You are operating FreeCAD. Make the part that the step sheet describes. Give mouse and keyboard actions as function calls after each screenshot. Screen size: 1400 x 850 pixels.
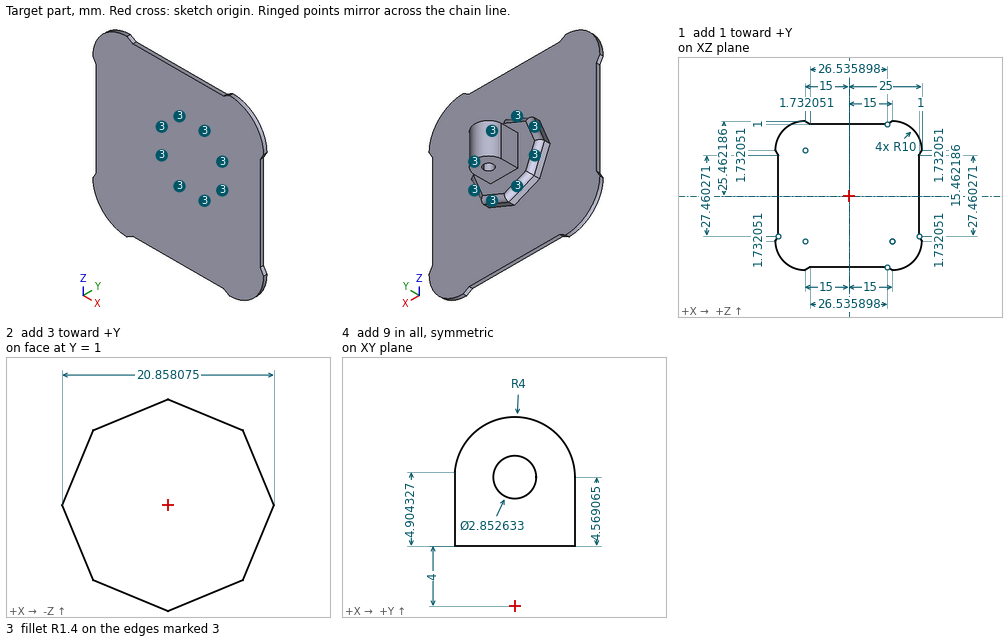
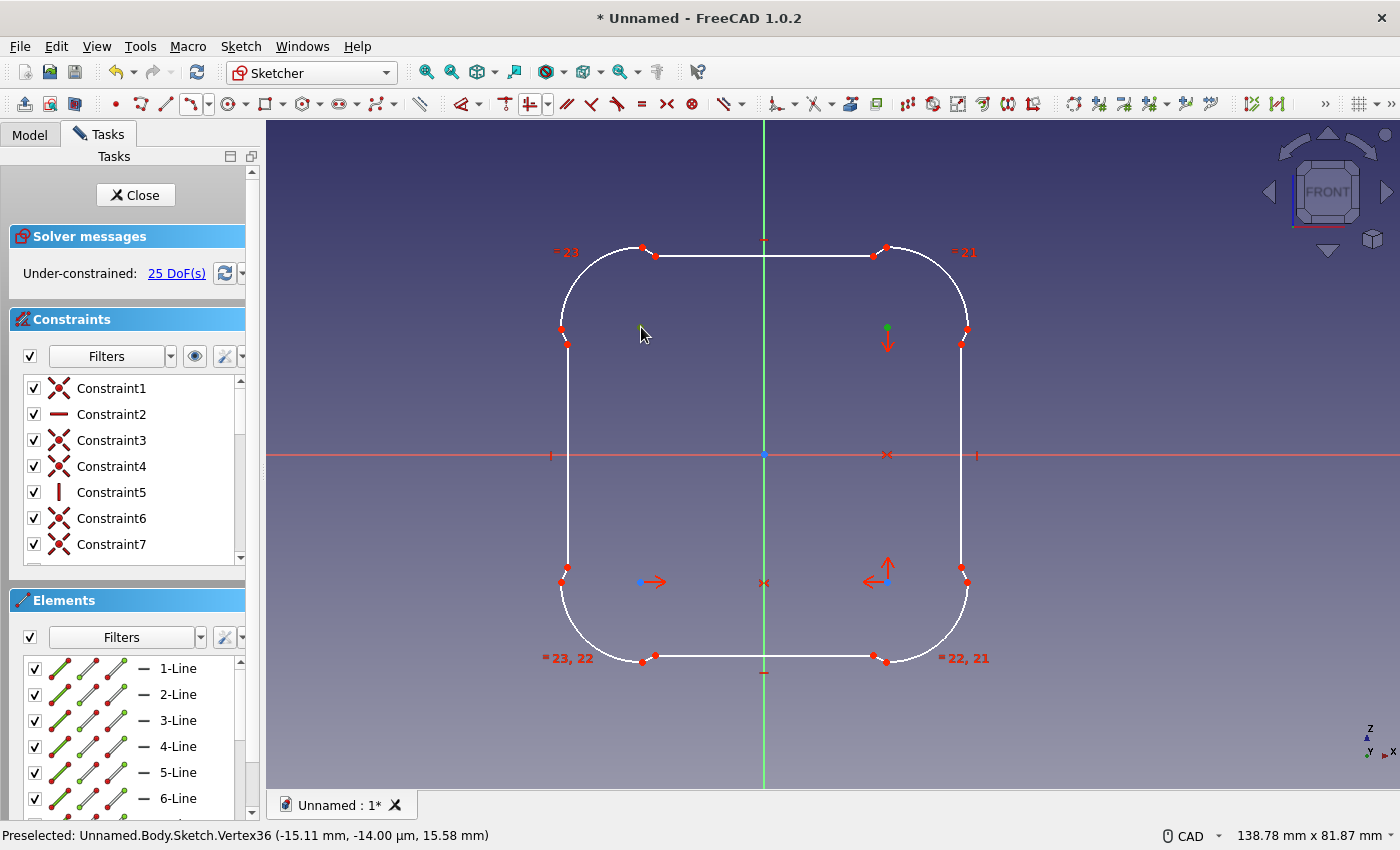
click(764, 717)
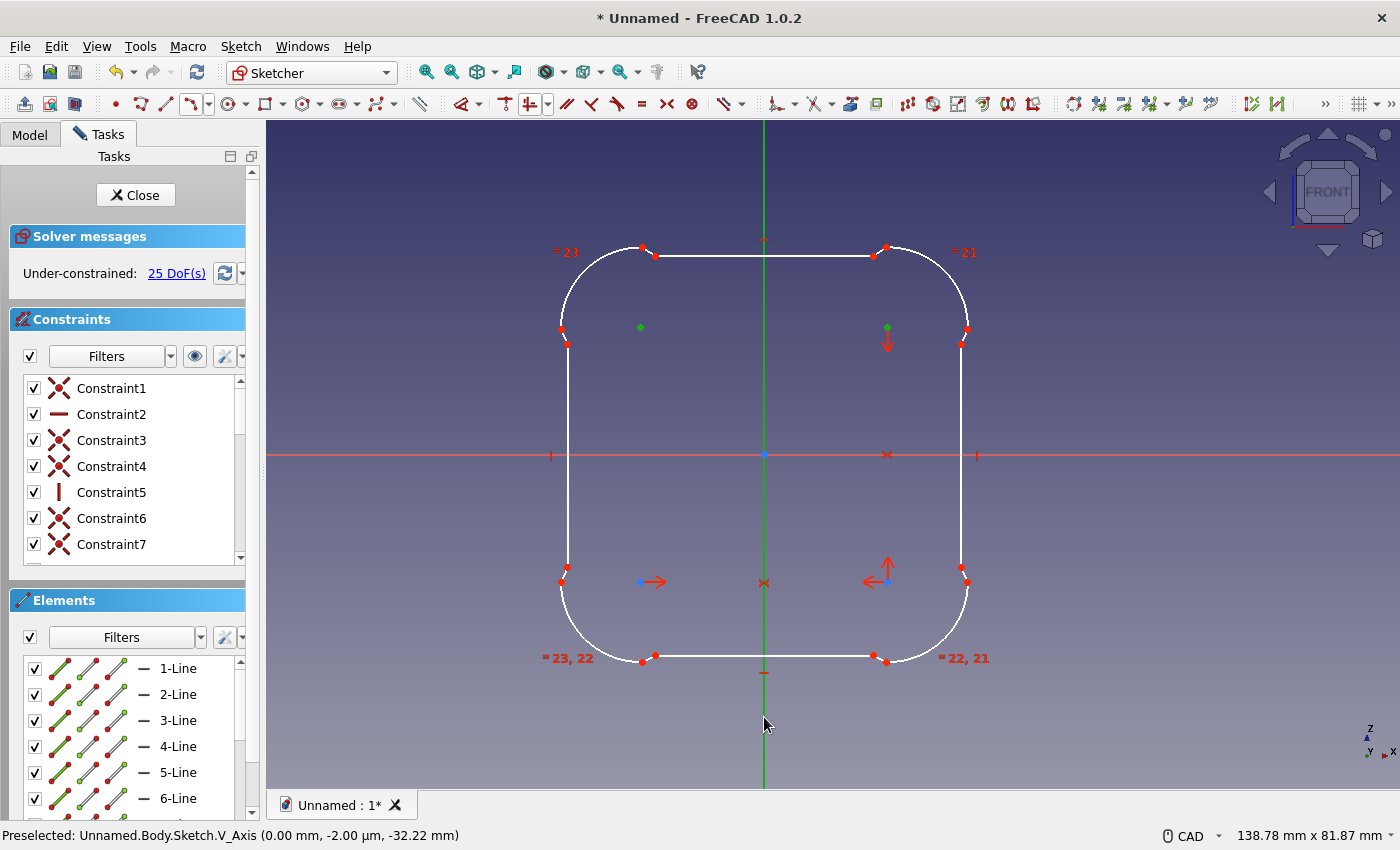
click(667, 104)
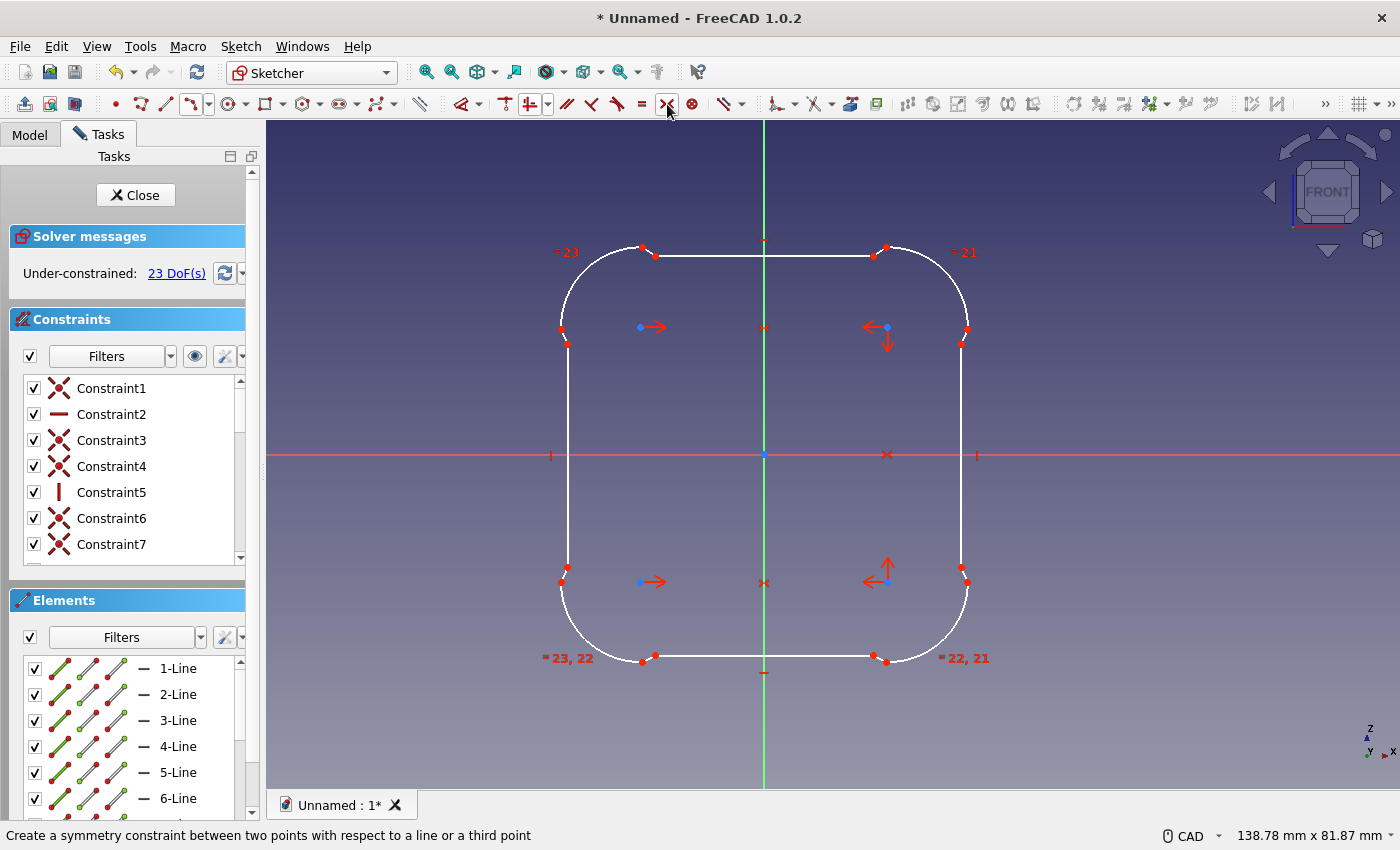
click(873, 256)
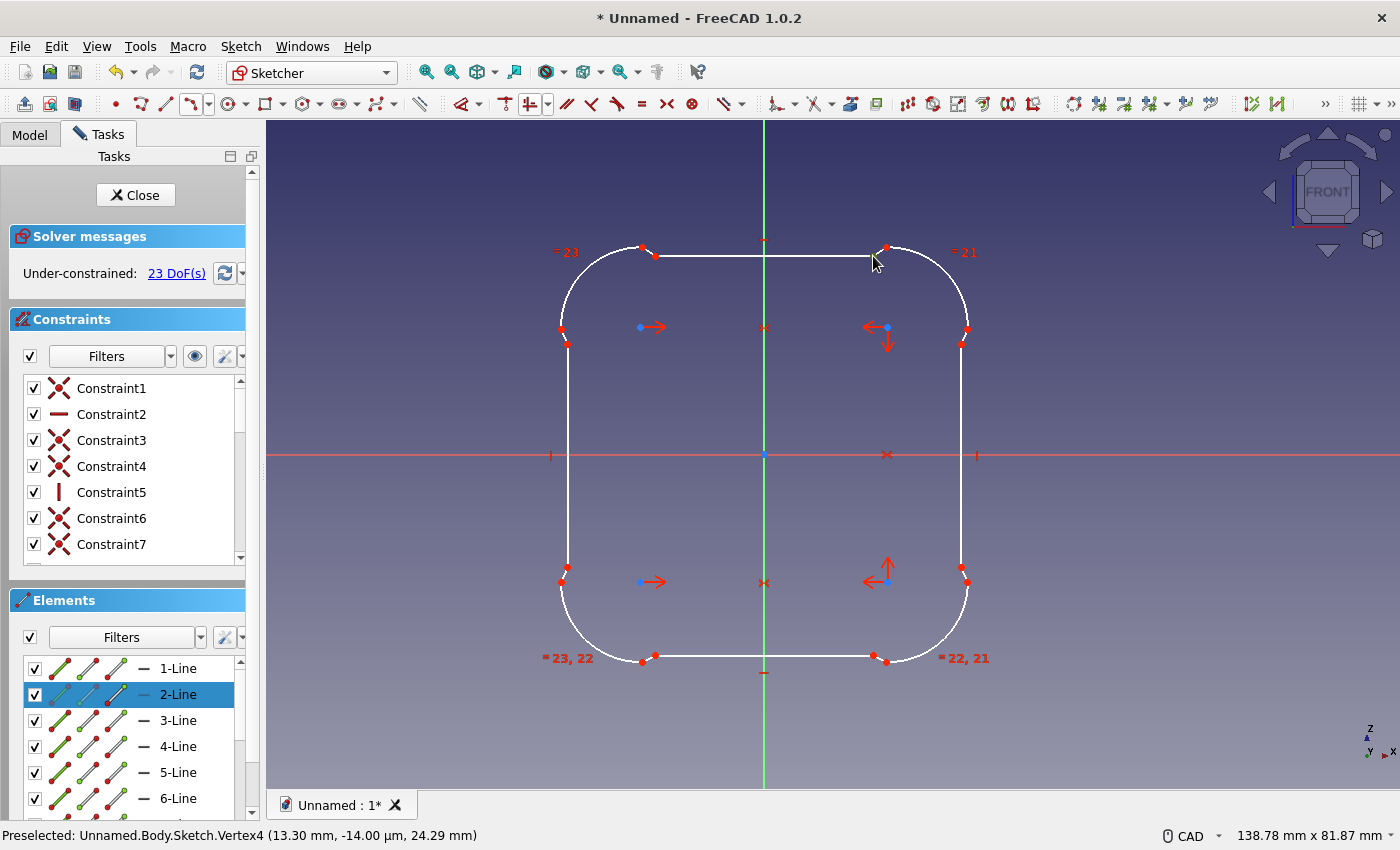
click(873, 656)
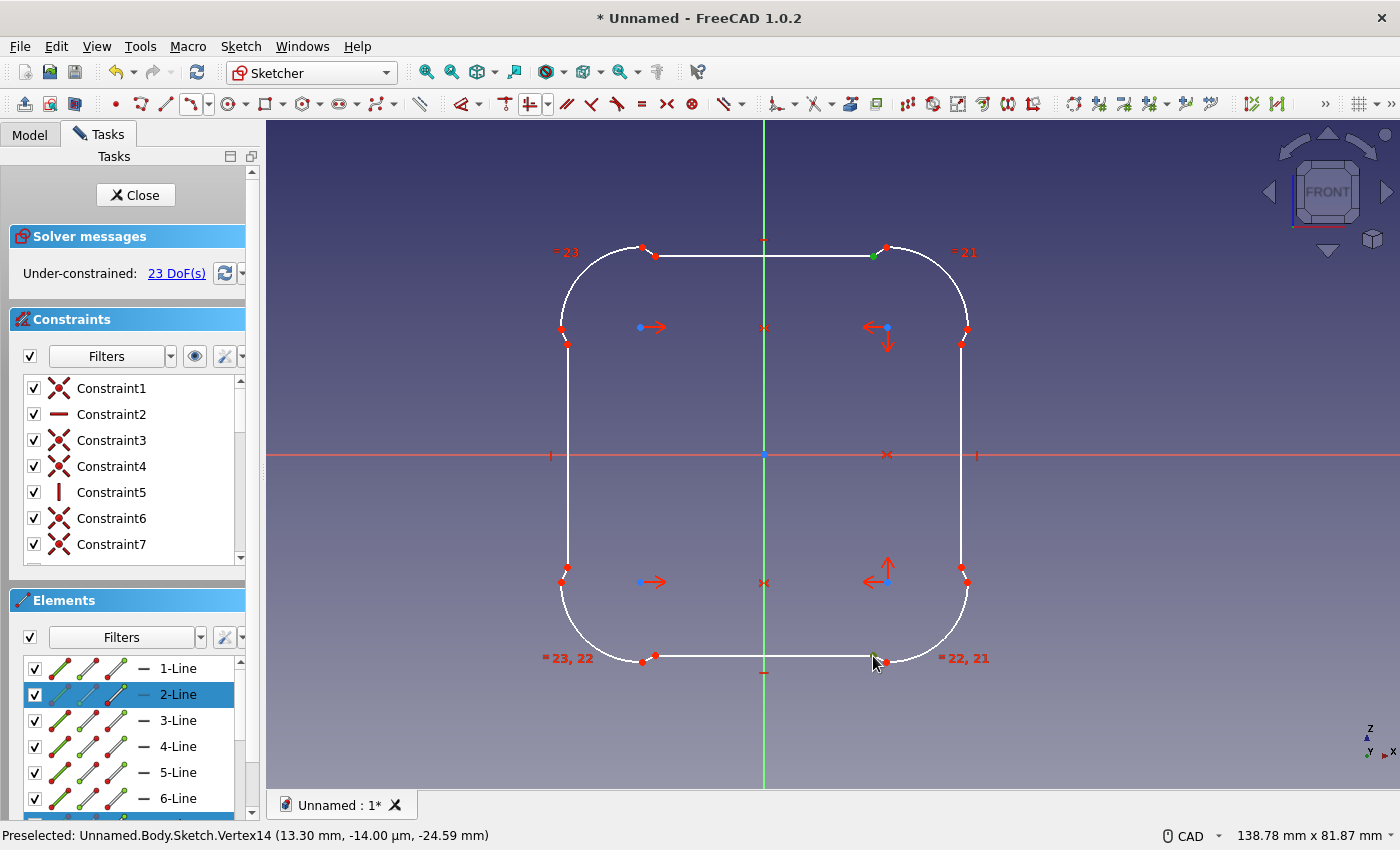
click(361, 455)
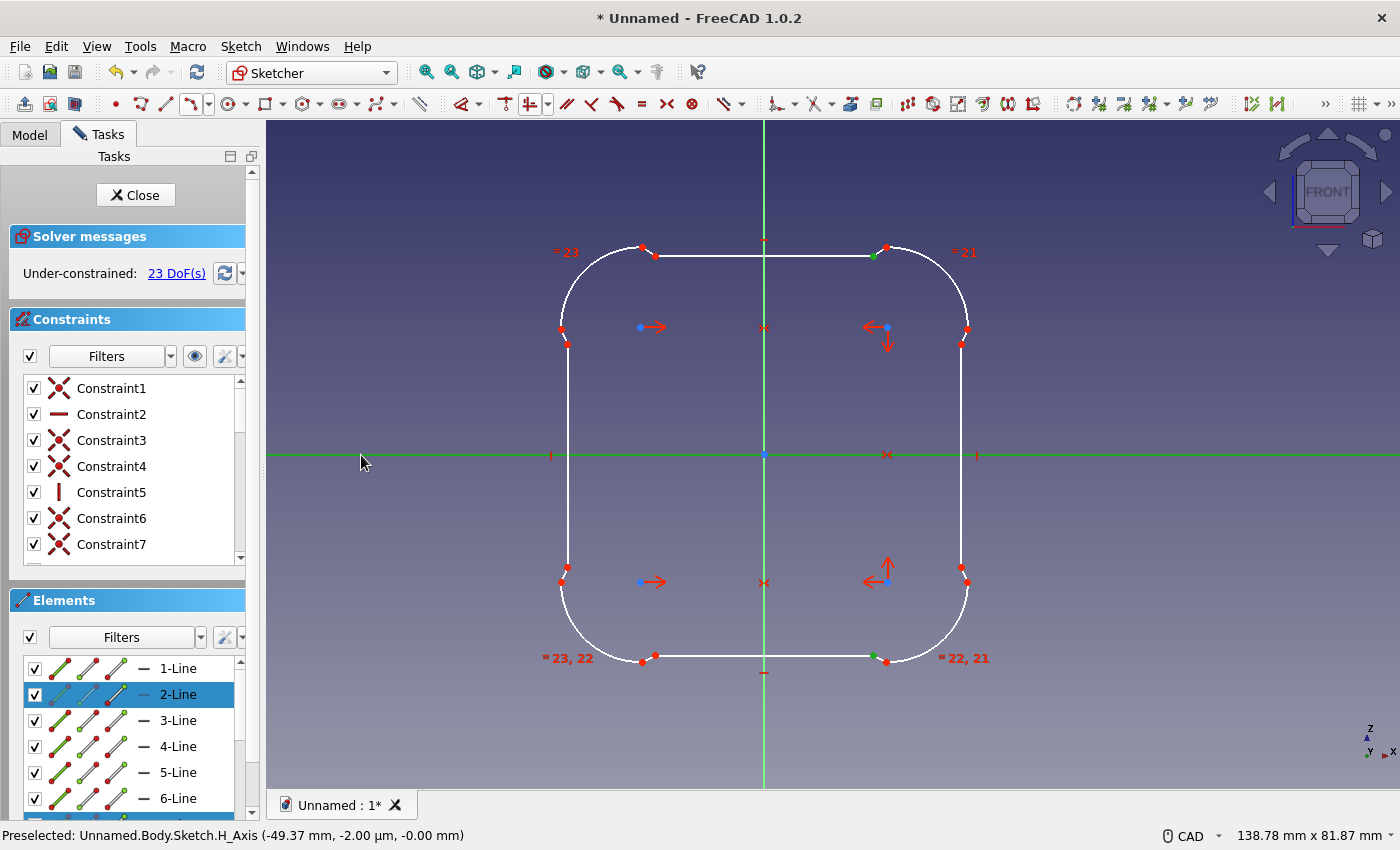
click(667, 104)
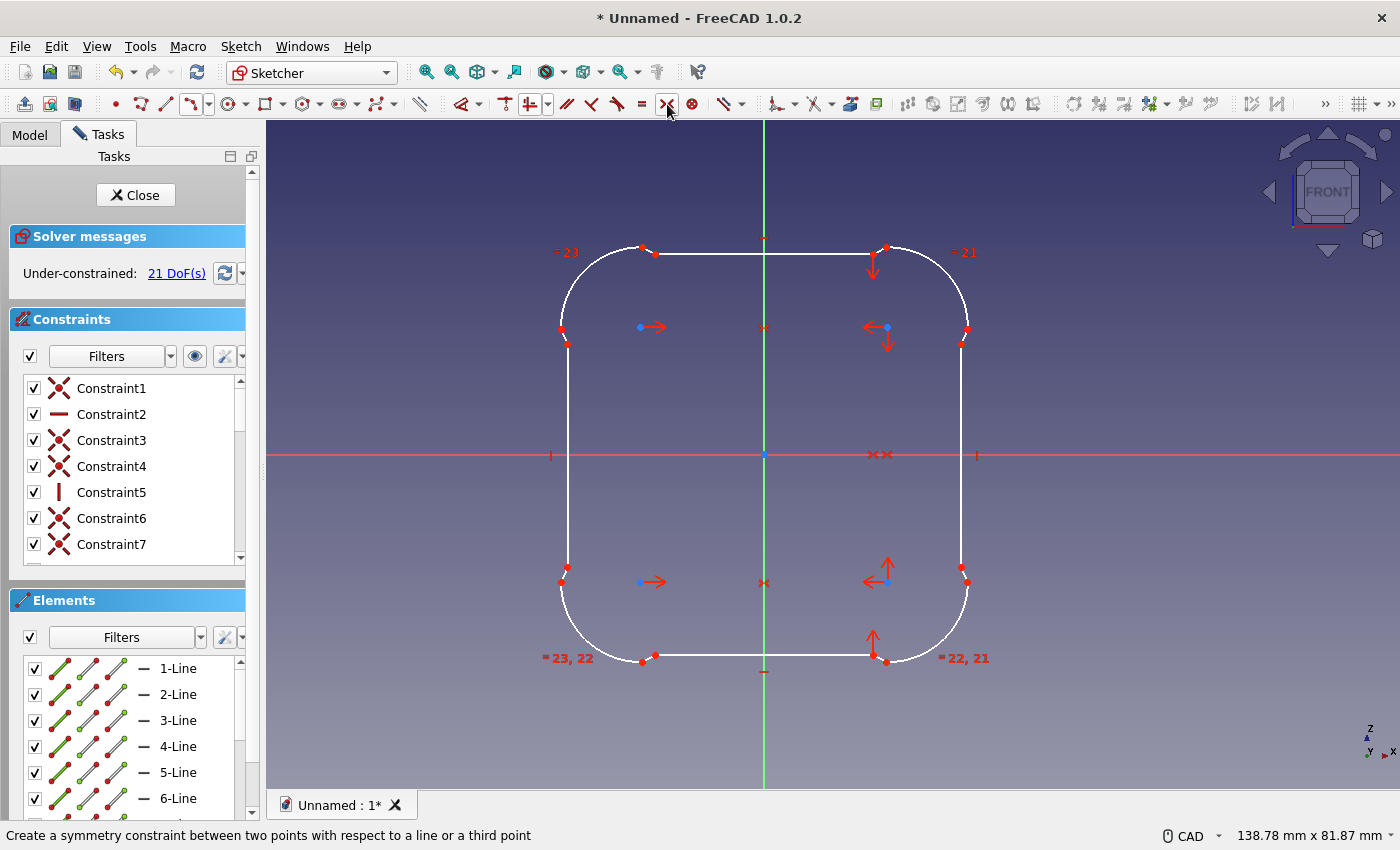
click(961, 568)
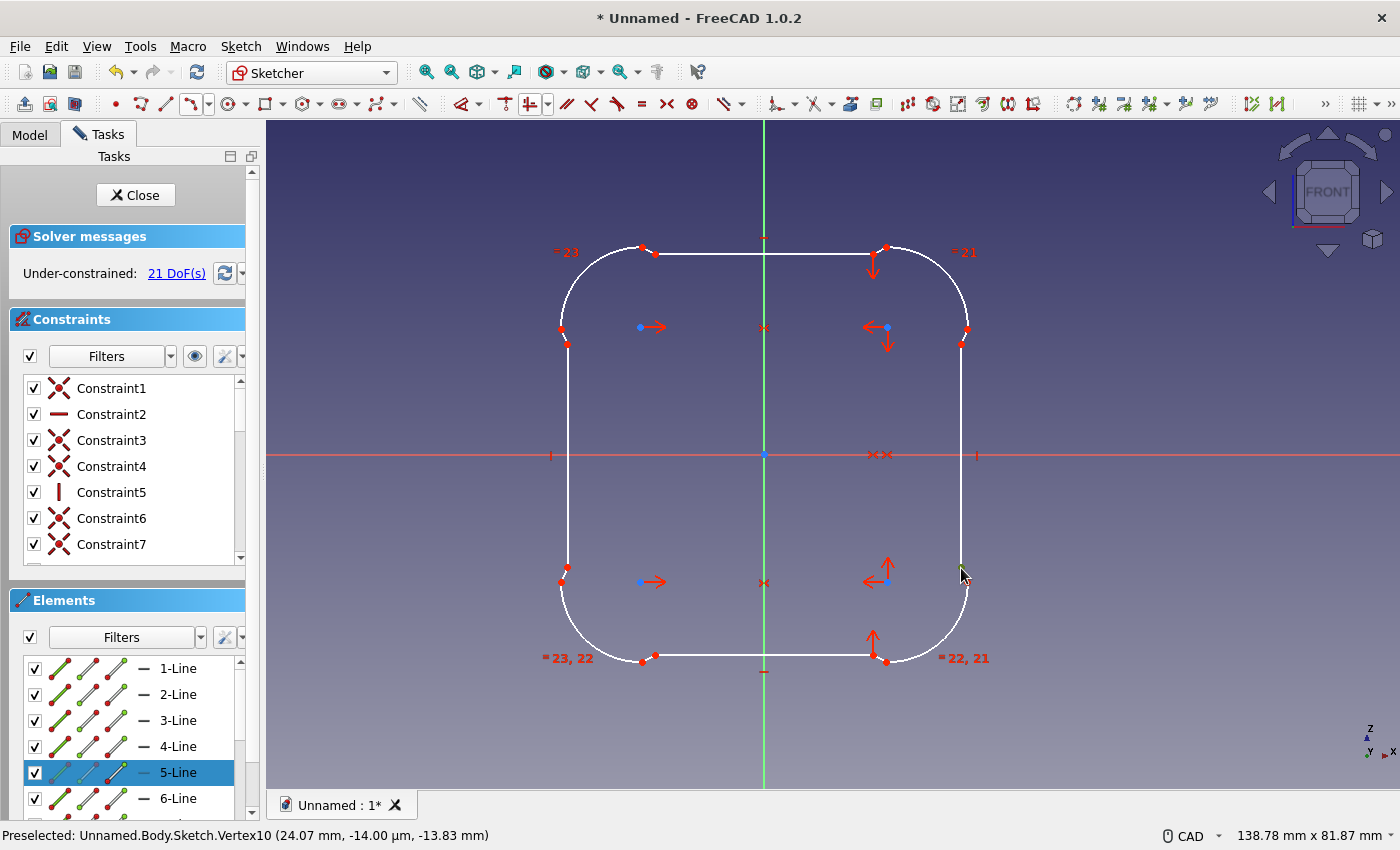
click(568, 568)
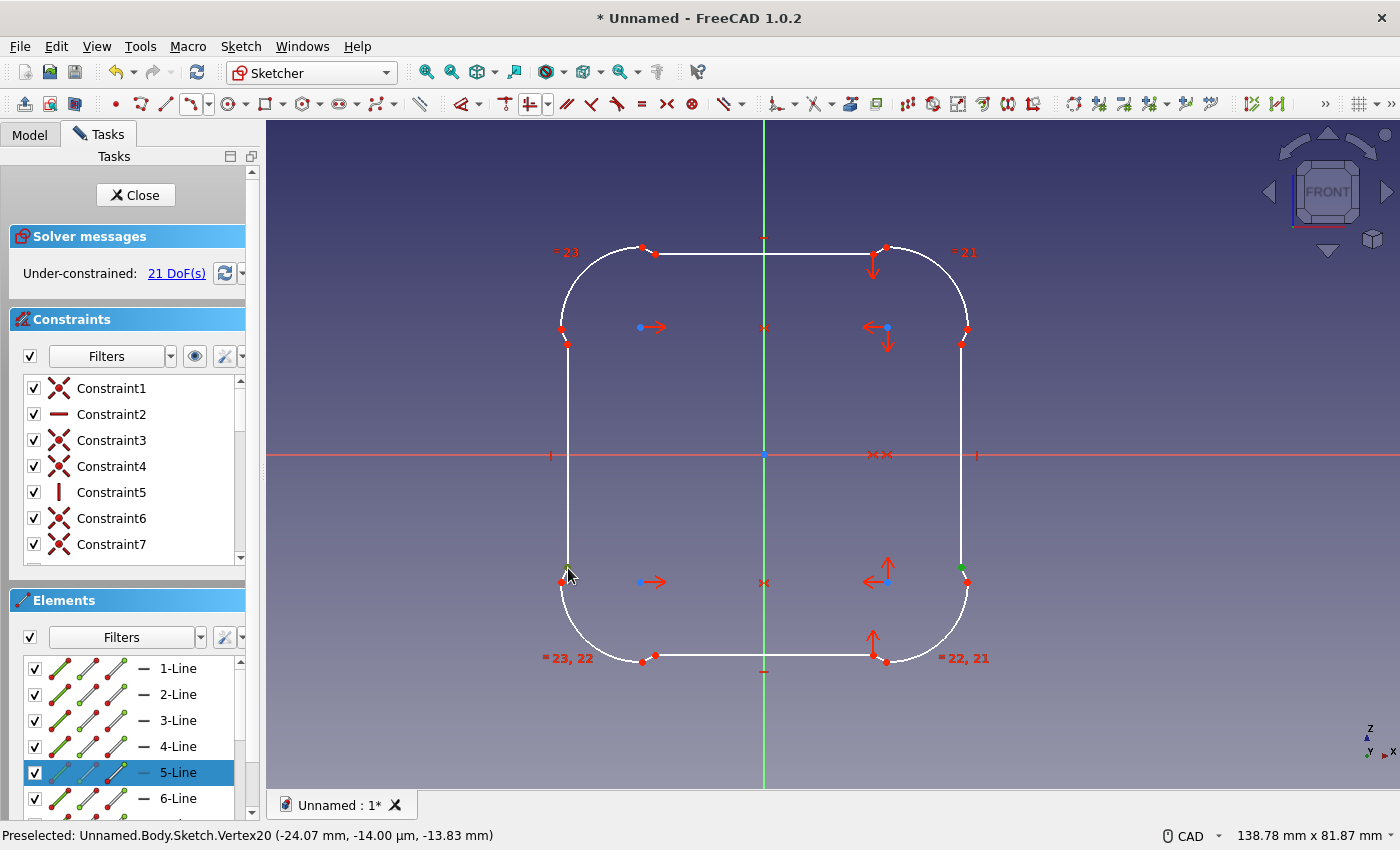
click(764, 717)